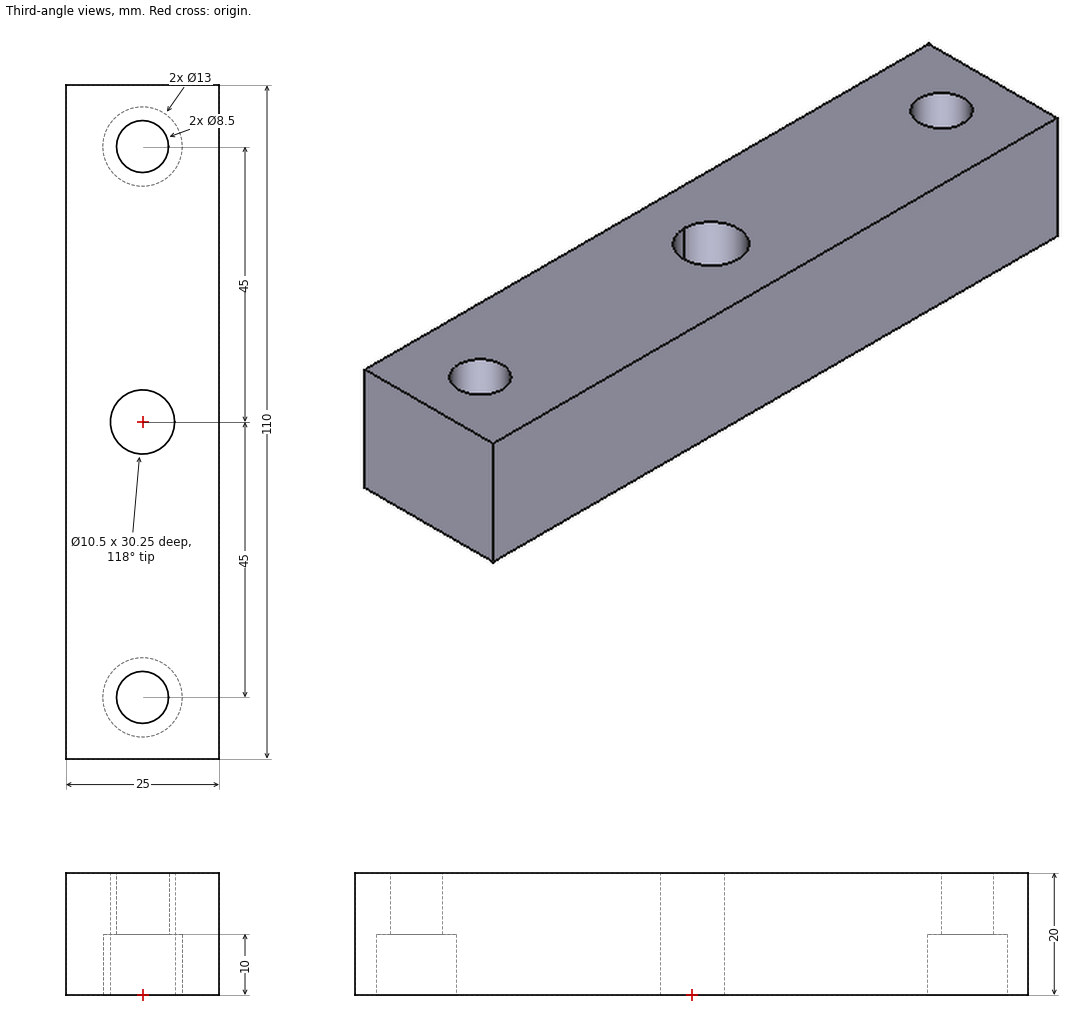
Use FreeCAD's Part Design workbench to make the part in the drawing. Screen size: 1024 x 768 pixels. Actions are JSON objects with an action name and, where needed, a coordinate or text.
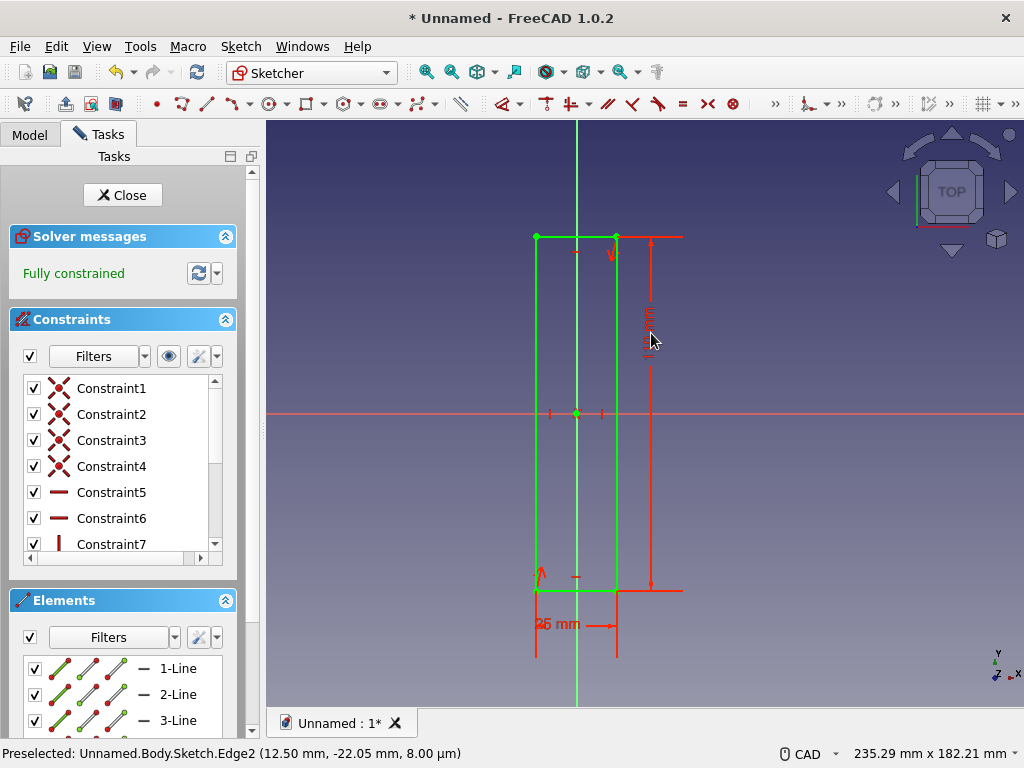
{"action": "left_click", "coordinate": [123, 195]}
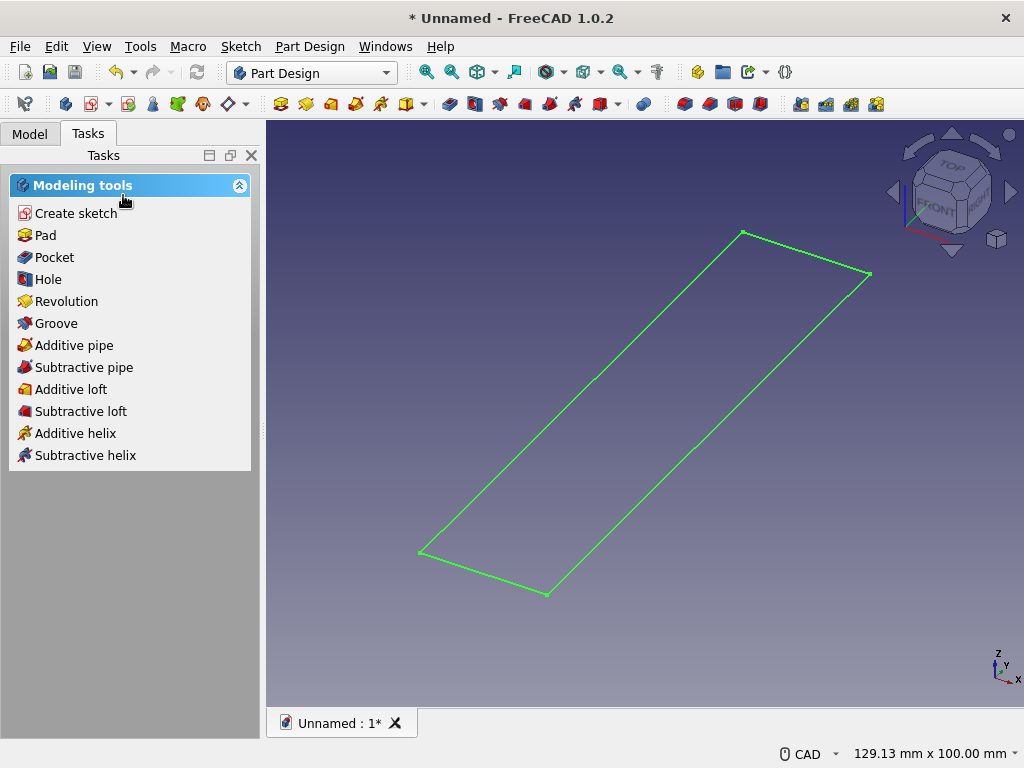
{"action": "left_click", "coordinate": [281, 104]}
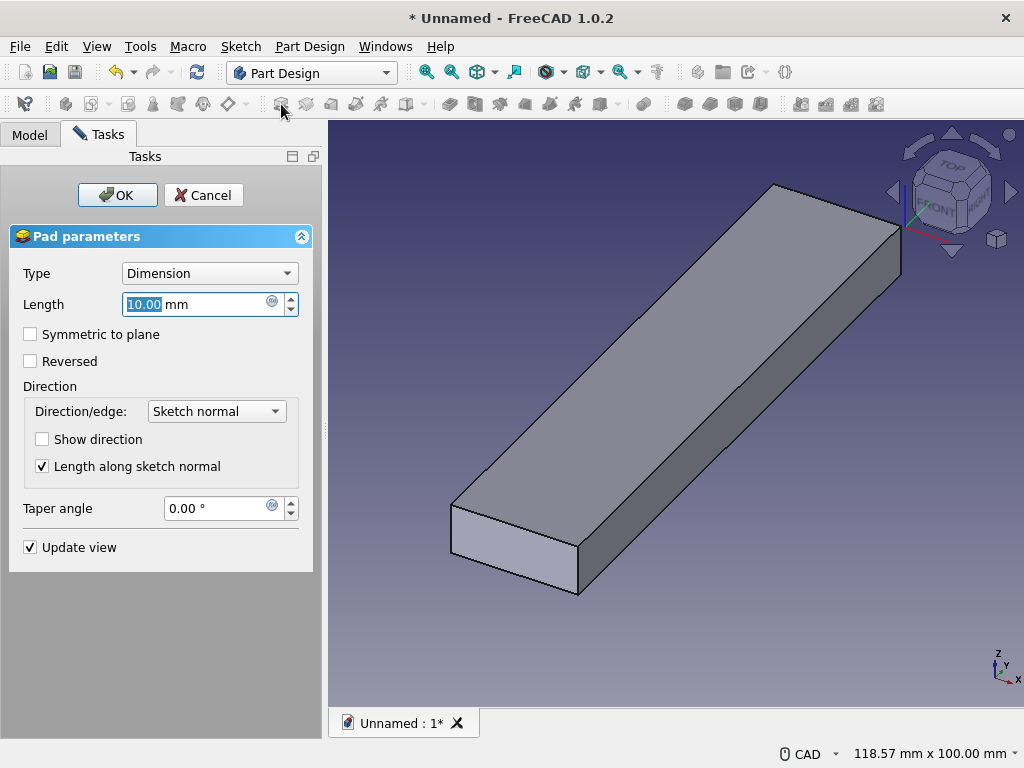
{"action": "type", "text": "20"}
{"action": "key", "text": "Tab"}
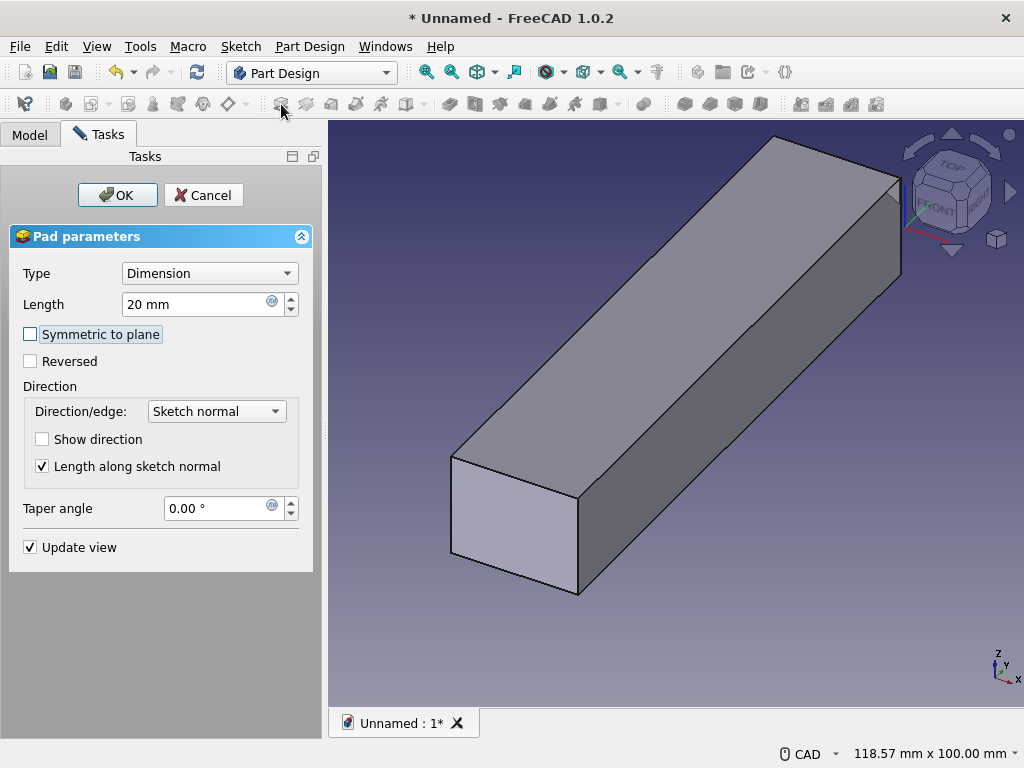
{"action": "left_click", "coordinate": [118, 195]}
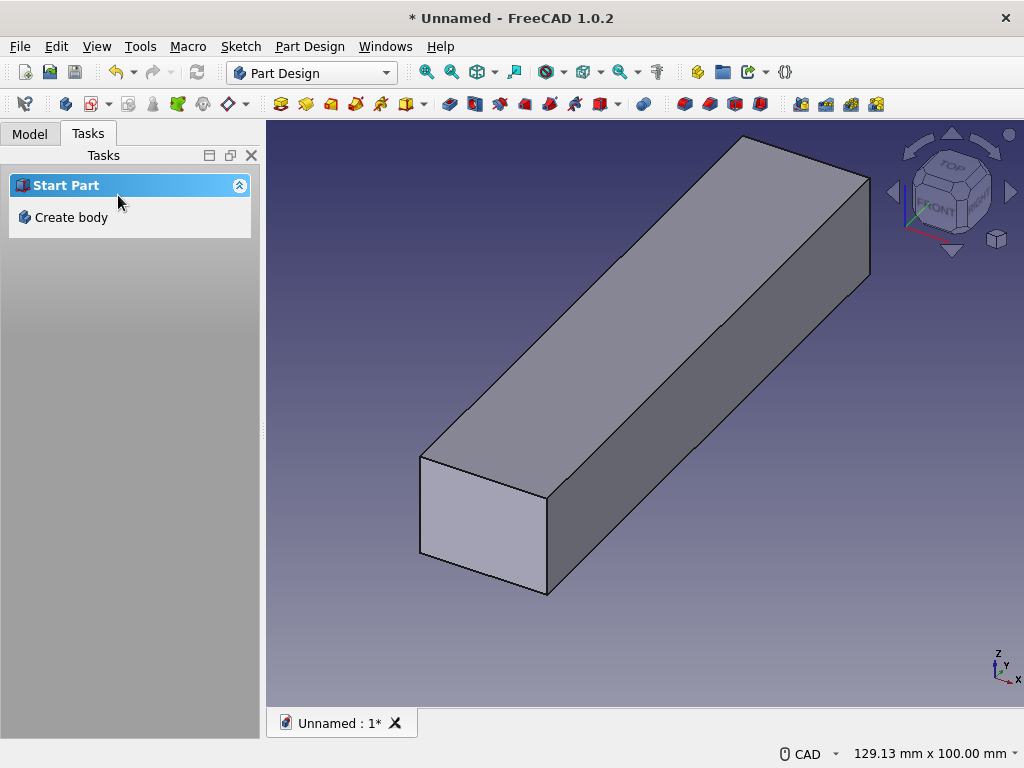
{"action": "left_click", "coordinate": [737, 225]}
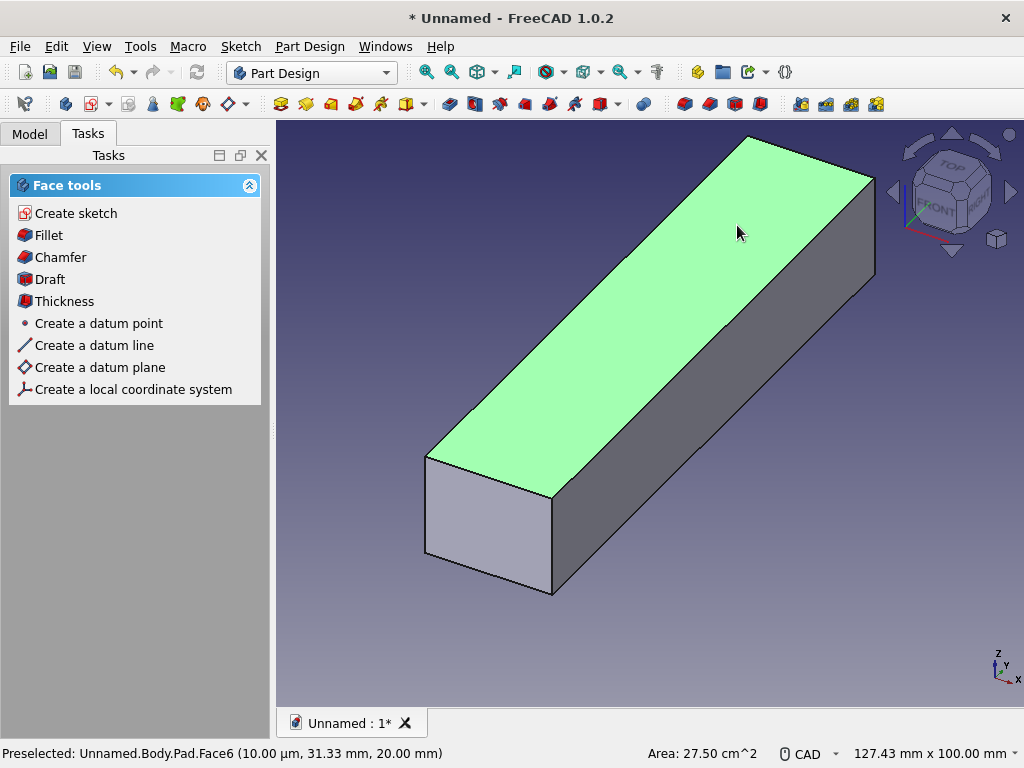
{"action": "left_click", "coordinate": [90, 104]}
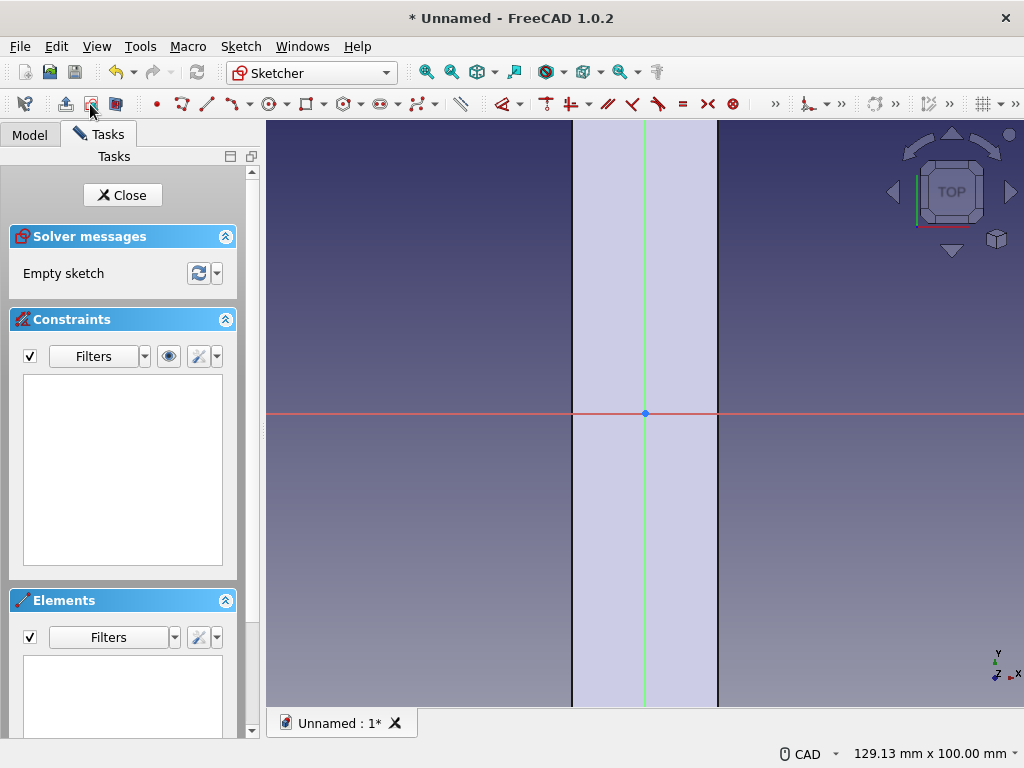
{"action": "scroll", "coordinate": [437, 414], "scroll_direction": "down", "scroll_amount": 2}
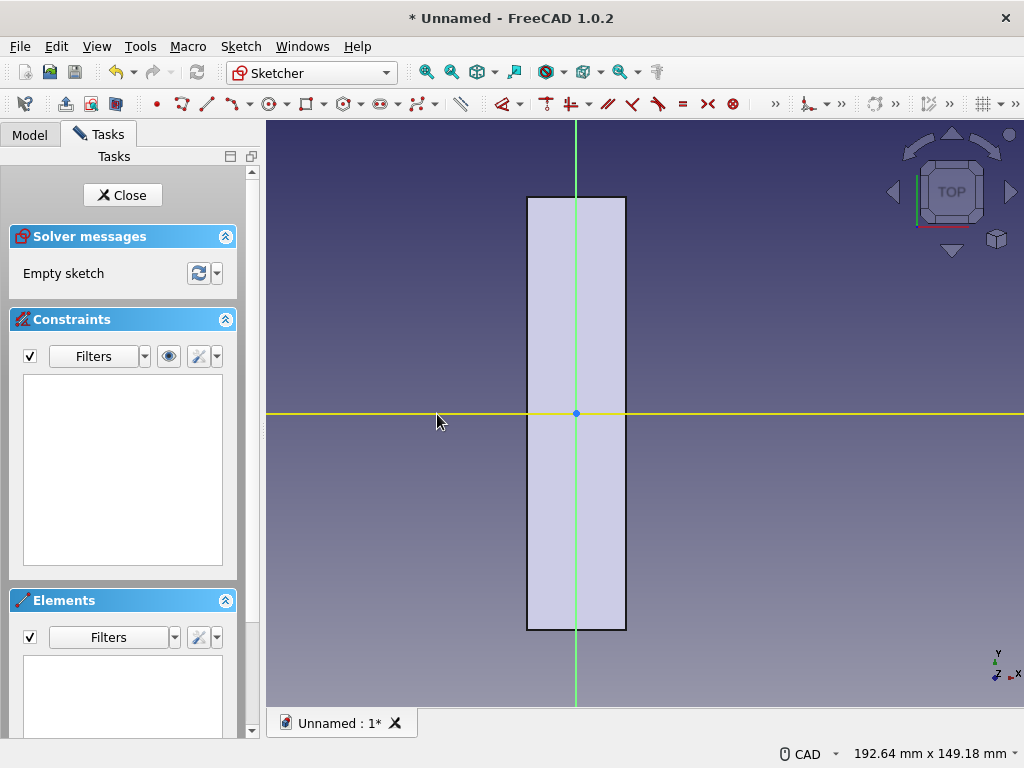
{"action": "left_click", "coordinate": [268, 104]}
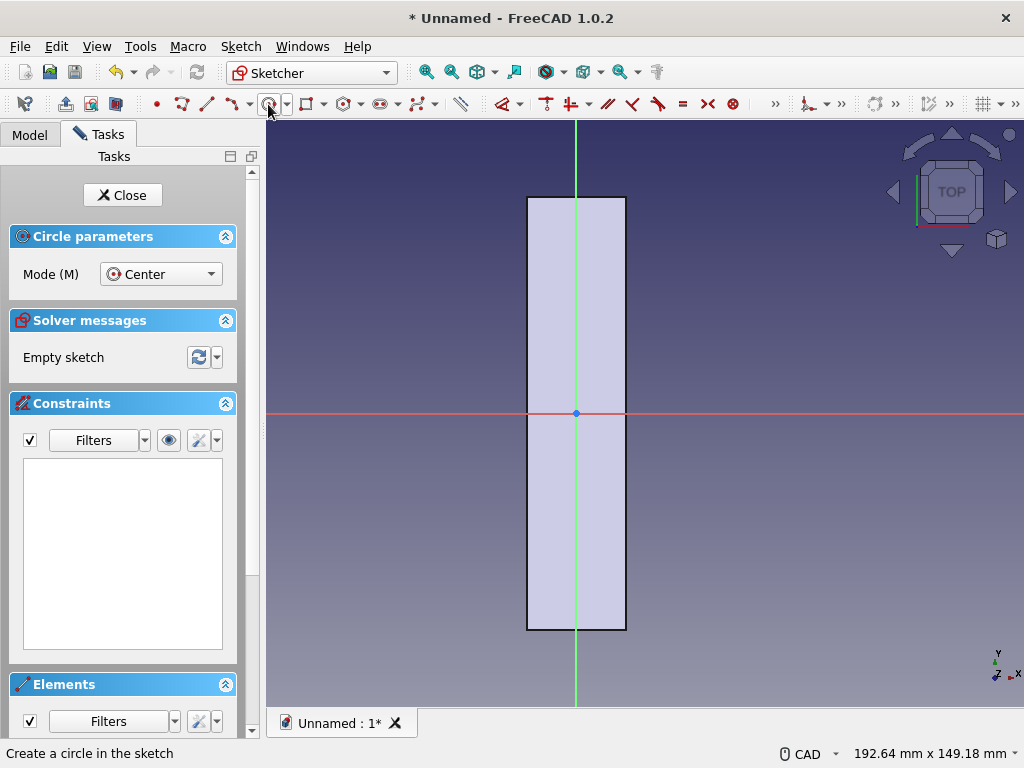
{"action": "scroll", "coordinate": [577, 237], "scroll_direction": "up", "scroll_amount": 2}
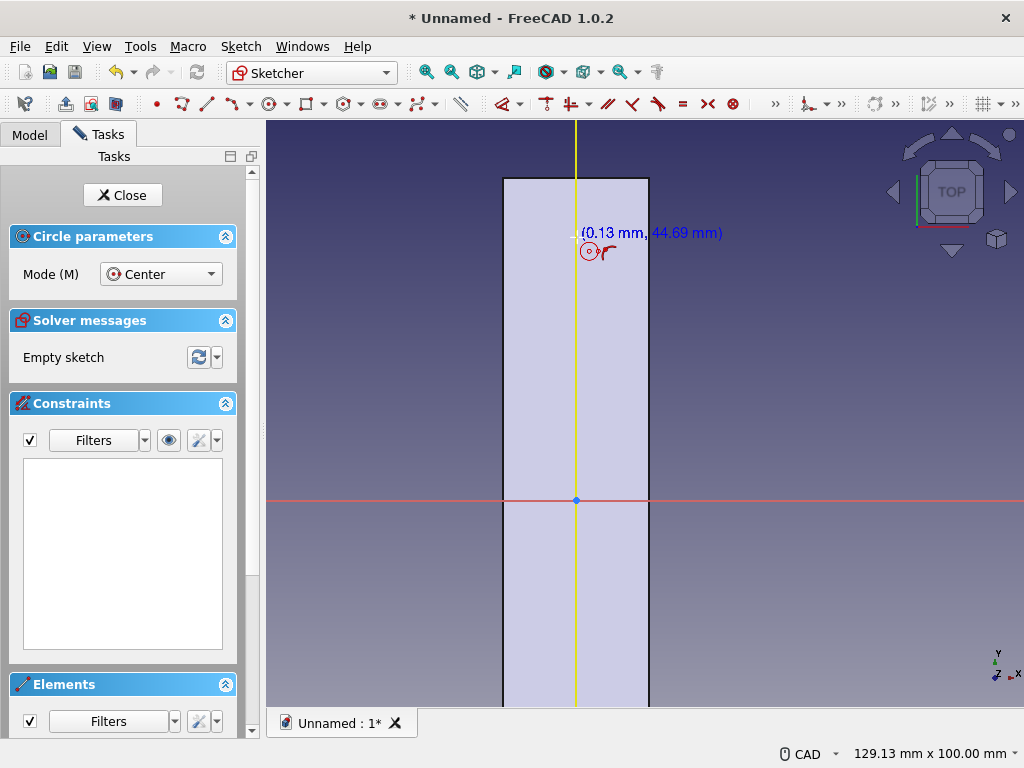
{"action": "left_click", "coordinate": [576, 237]}
{"action": "left_click", "coordinate": [594, 219]}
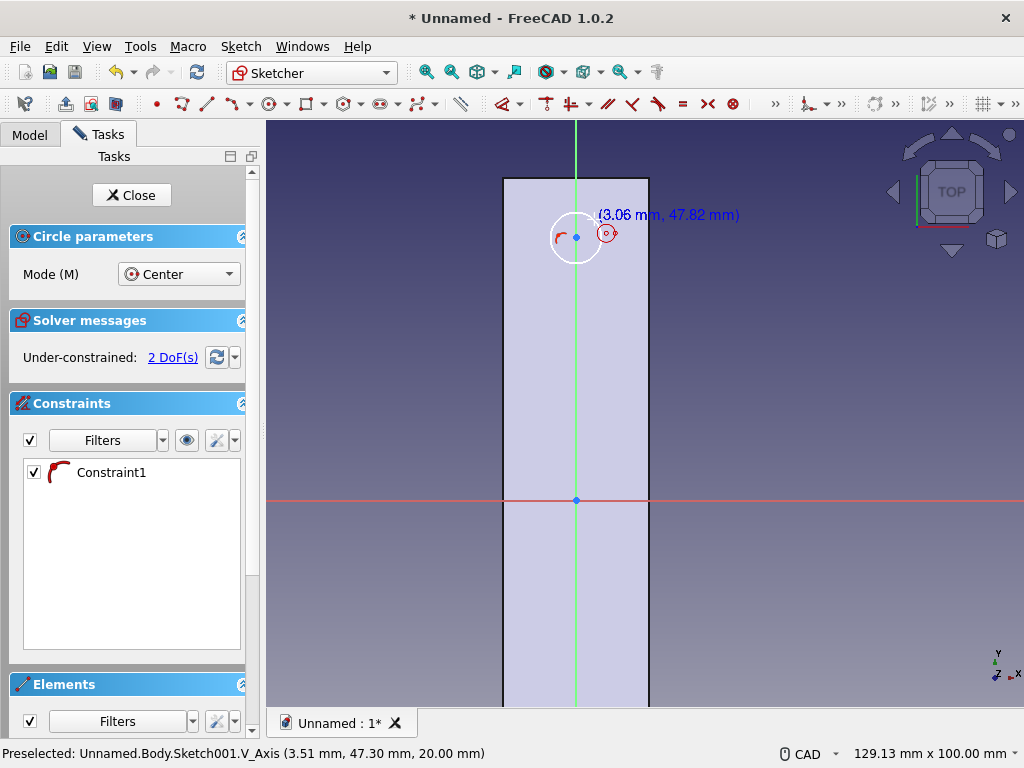
{"action": "scroll", "coordinate": [577, 236], "scroll_direction": "down", "scroll_amount": 2}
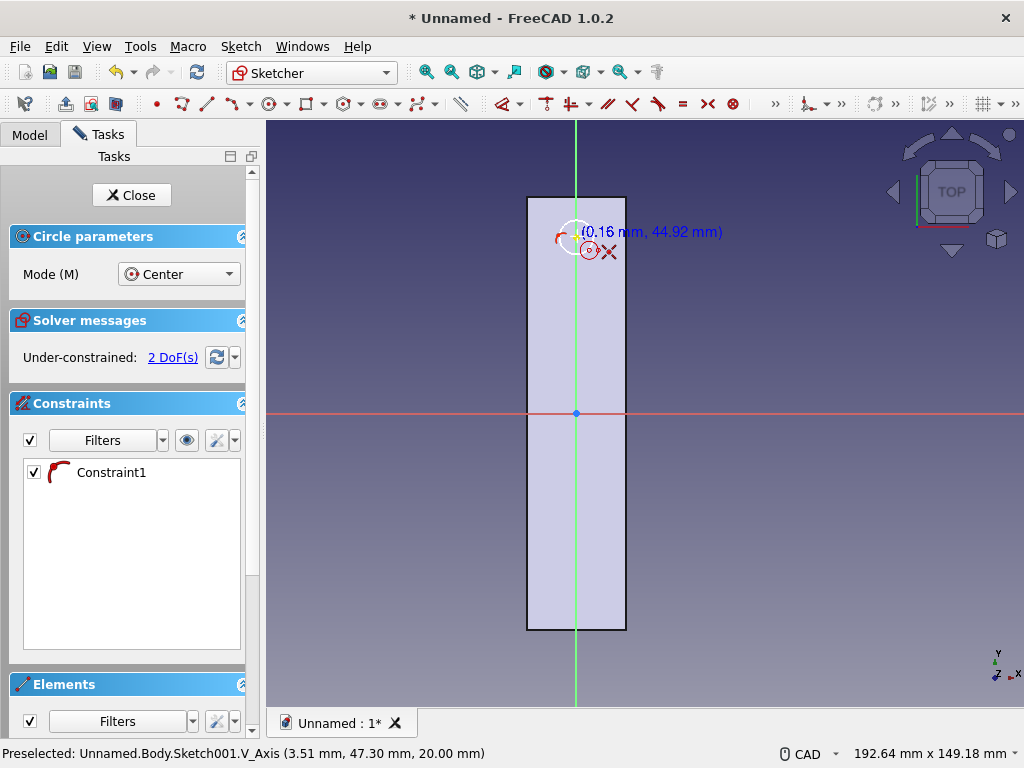
{"action": "scroll", "coordinate": [577, 591], "scroll_direction": "up", "scroll_amount": 2}